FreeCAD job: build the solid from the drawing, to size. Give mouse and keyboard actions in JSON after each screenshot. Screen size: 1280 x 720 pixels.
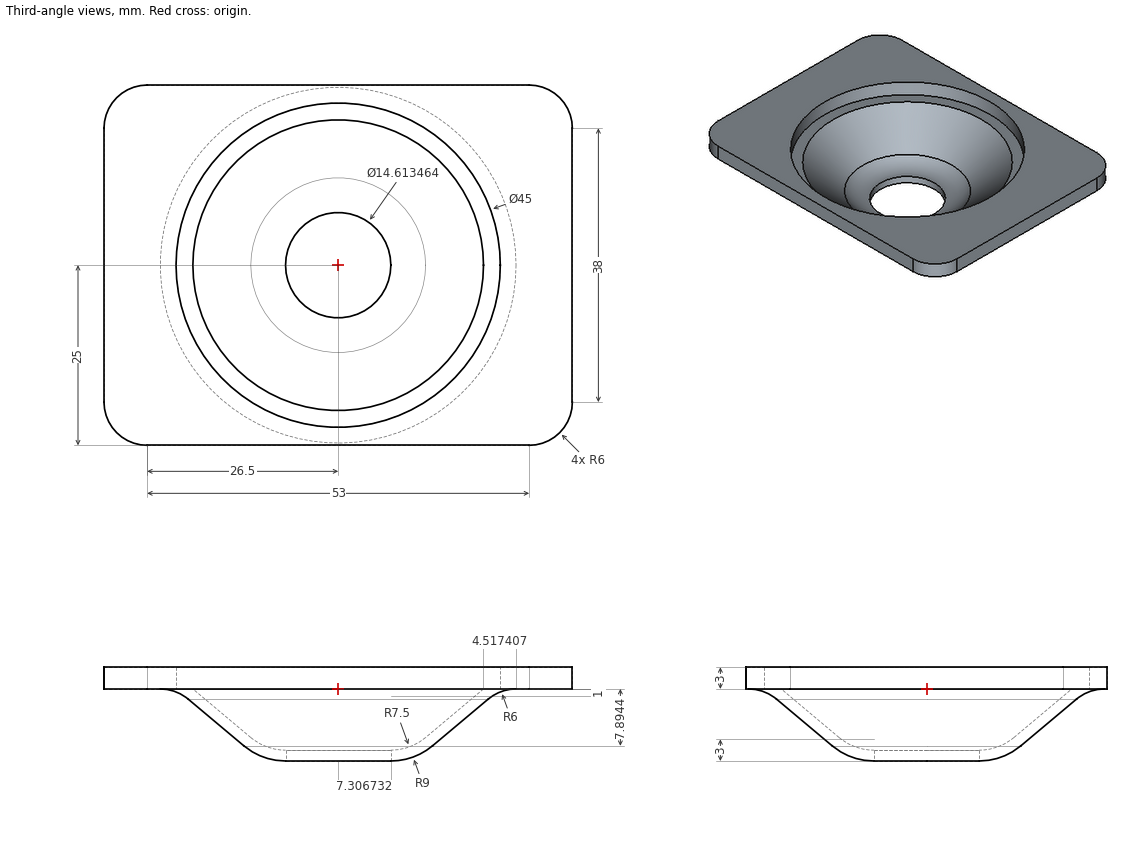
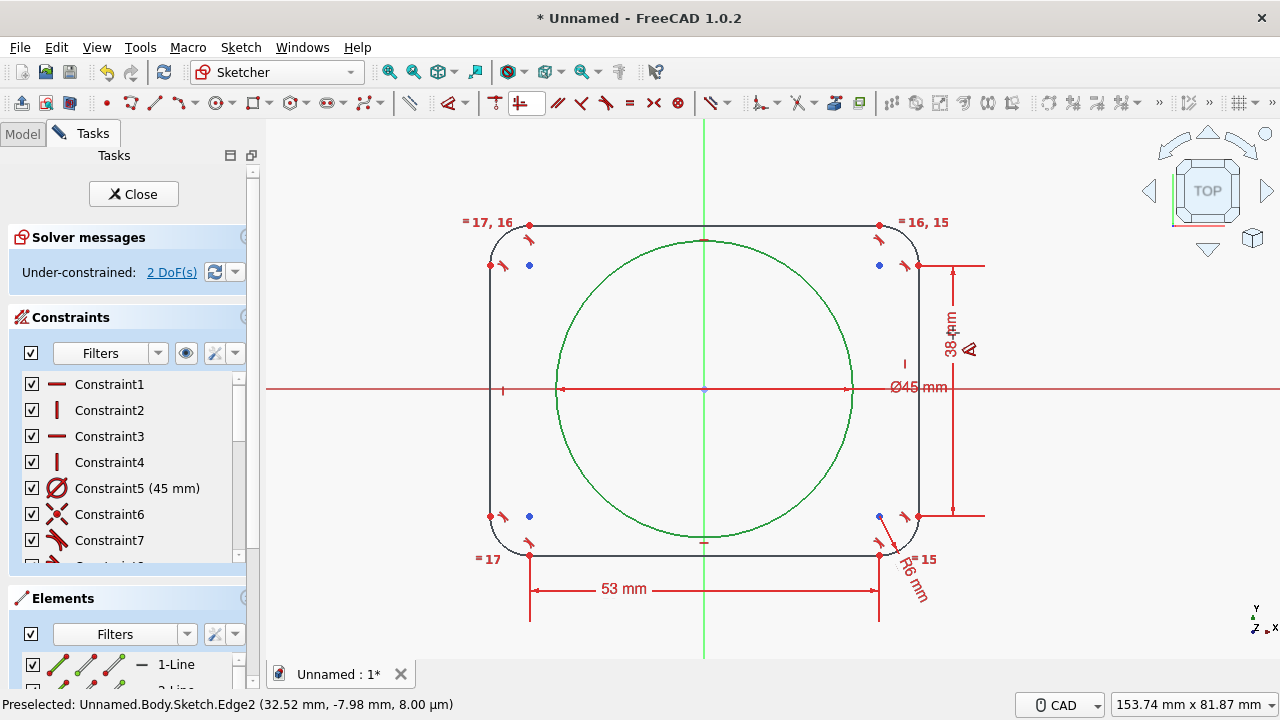
{"action": "left_click", "coordinate": [530, 556]}
{"action": "left_click", "coordinate": [738, 473]}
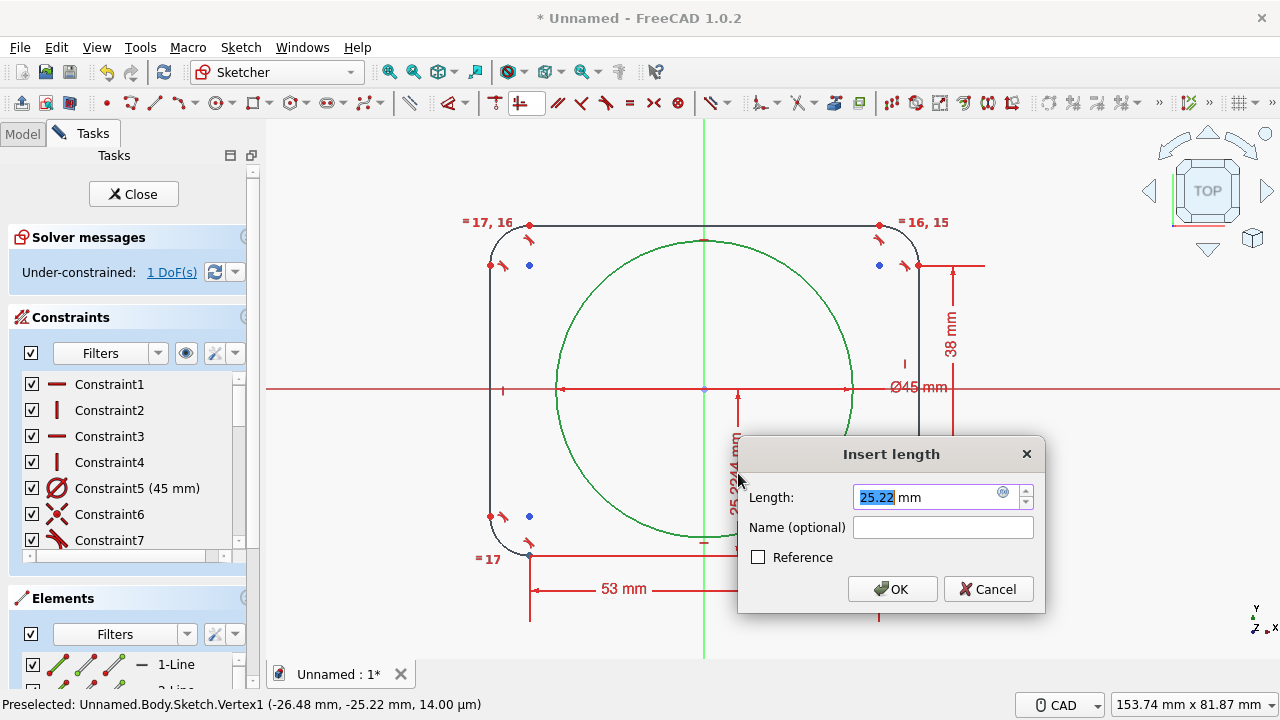
{"action": "type", "text": "25"}
{"action": "key", "text": "Return"}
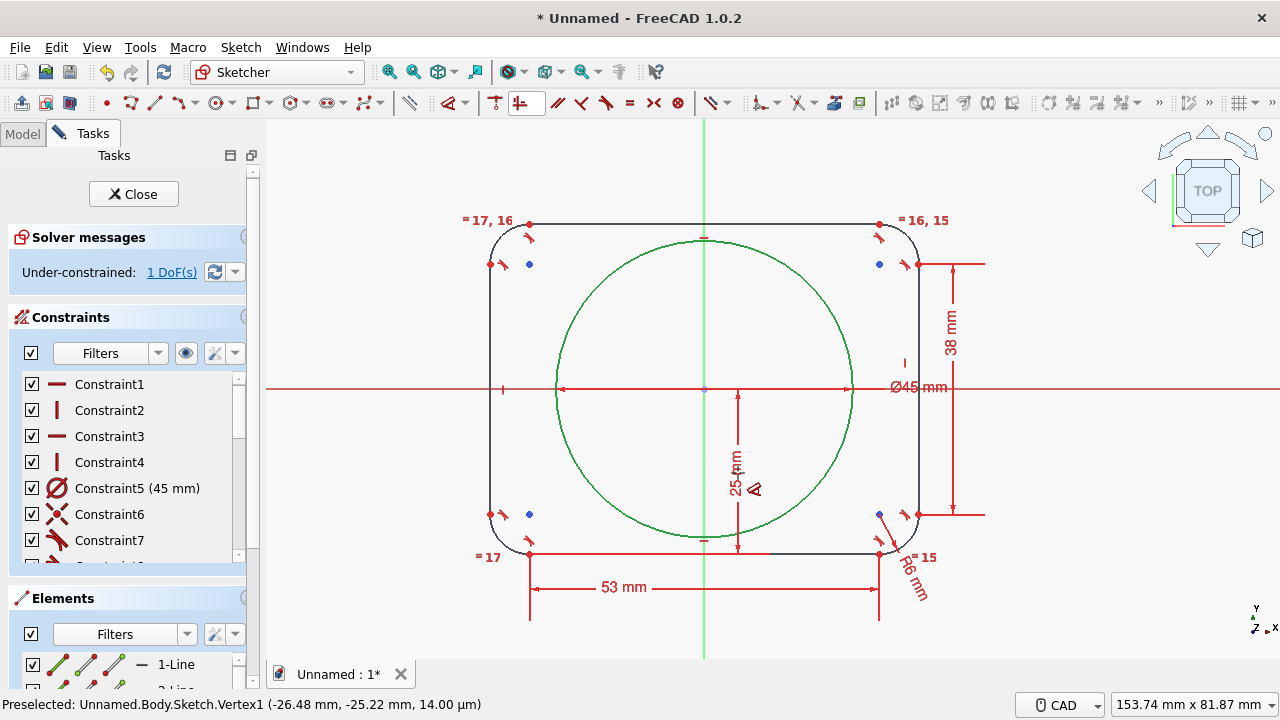
{"action": "left_click", "coordinate": [530, 554]}
{"action": "left_click", "coordinate": [617, 355]}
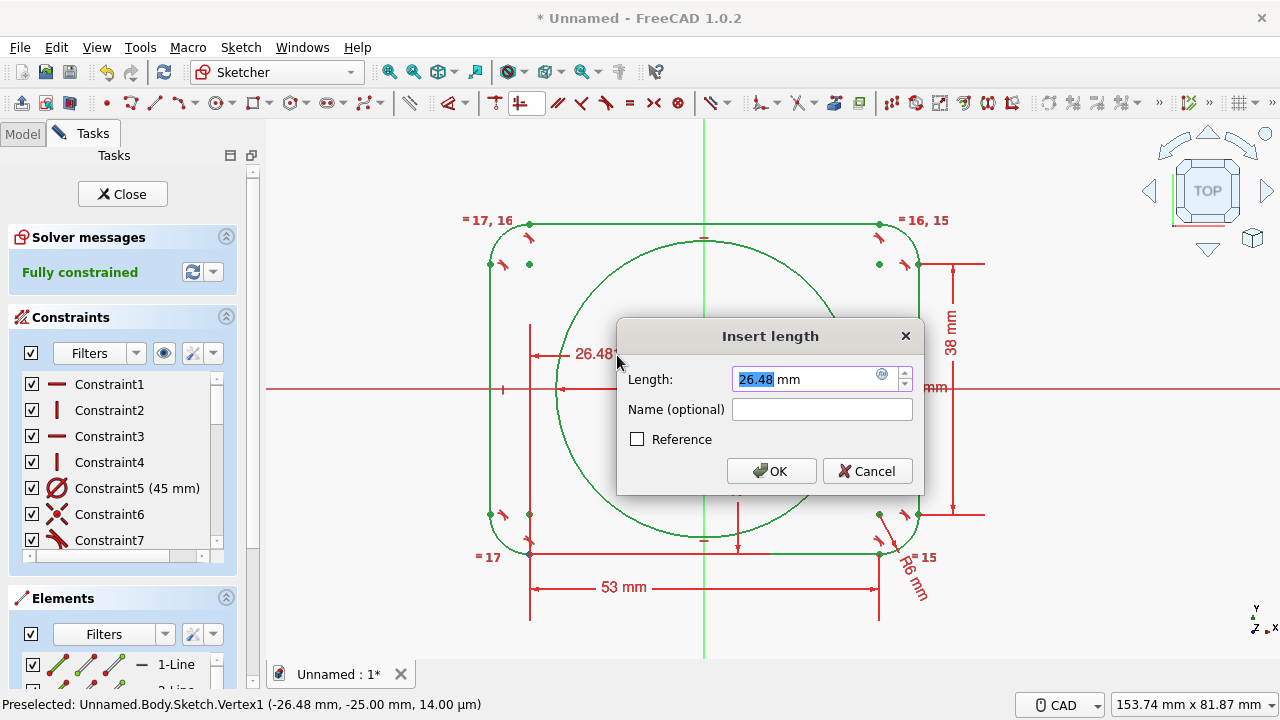
{"action": "type", "text": "26.5"}
{"action": "key", "text": "Return"}
{"action": "key", "text": "Escape"}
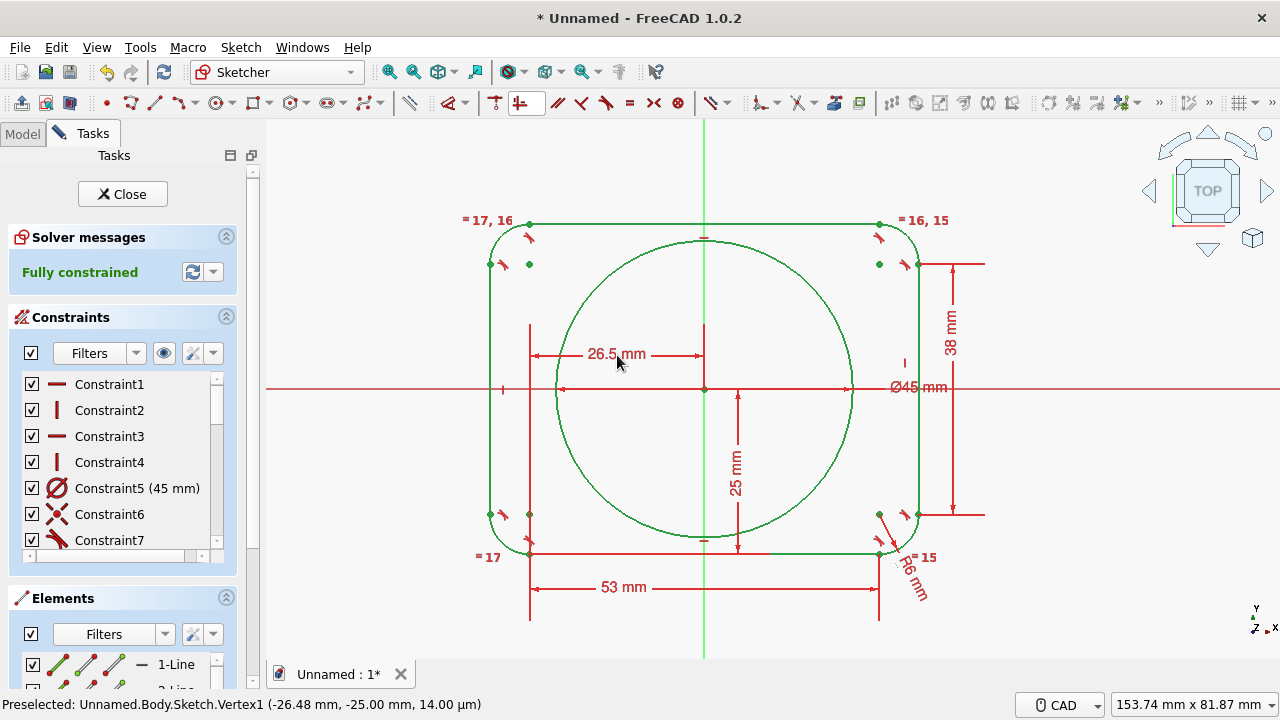
{"action": "left_click", "coordinate": [123, 194]}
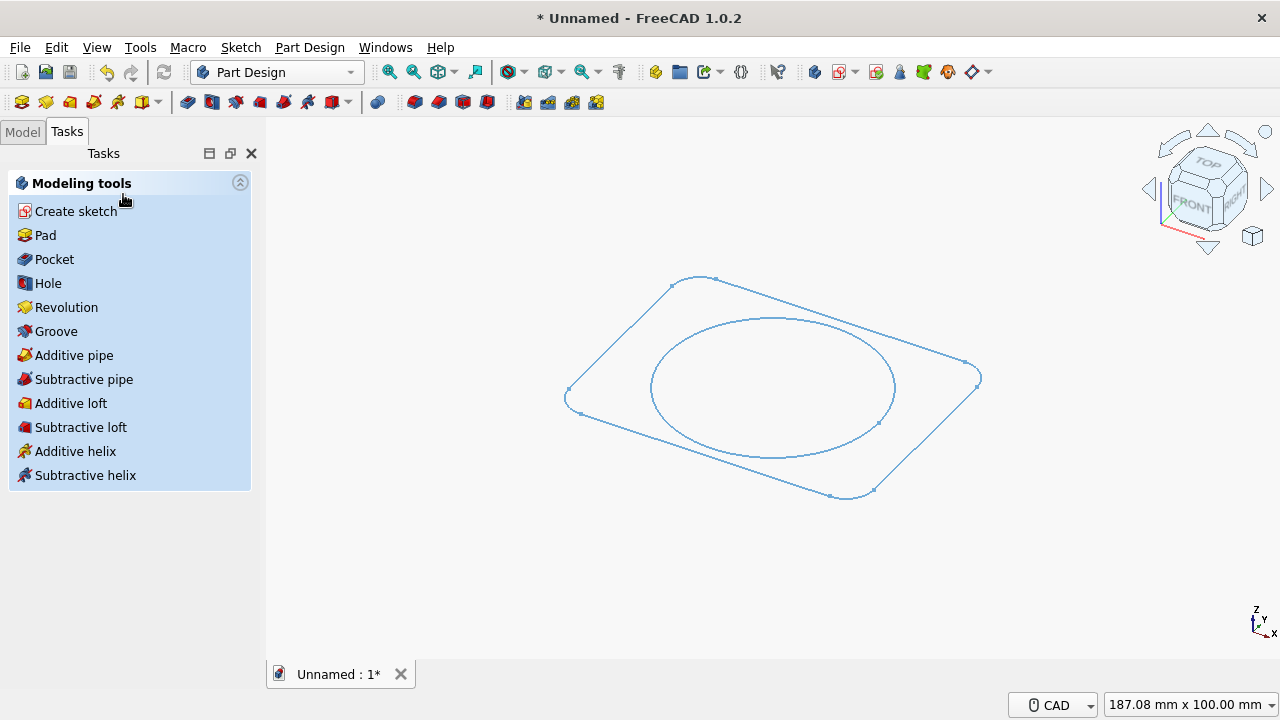
{"action": "left_click", "coordinate": [22, 102]}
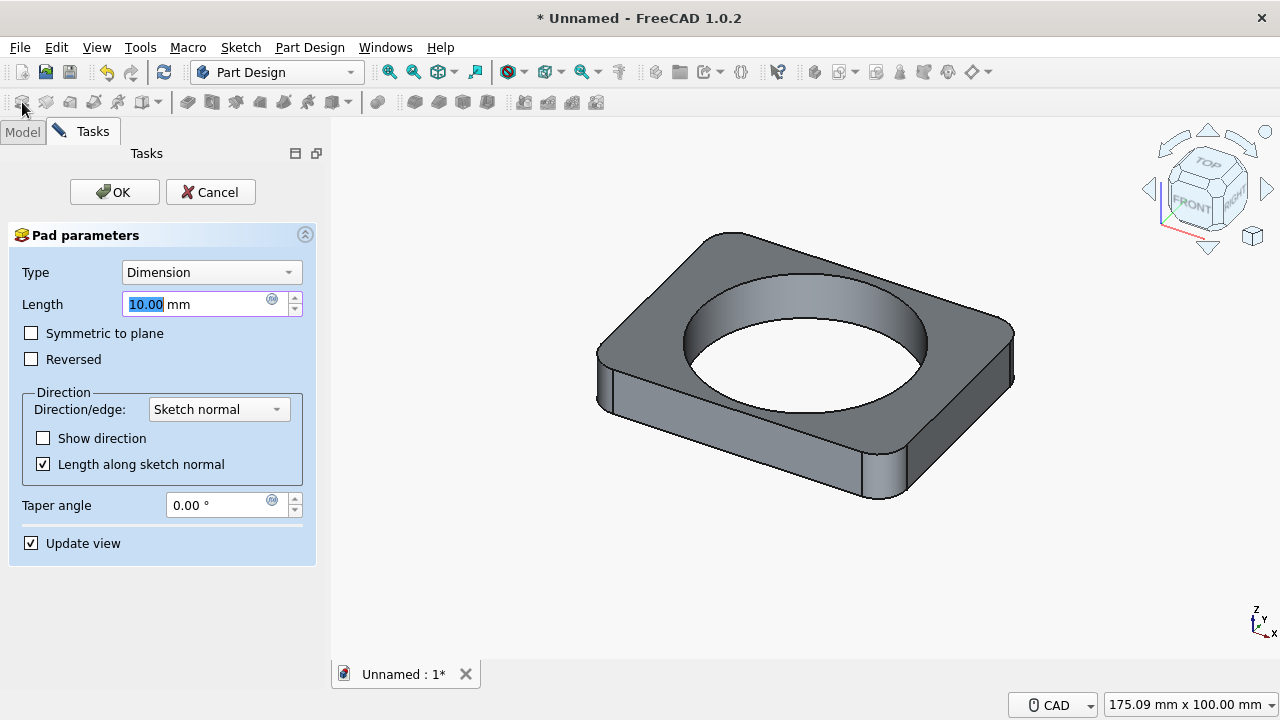
{"action": "type", "text": "3"}
{"action": "key", "text": "Tab"}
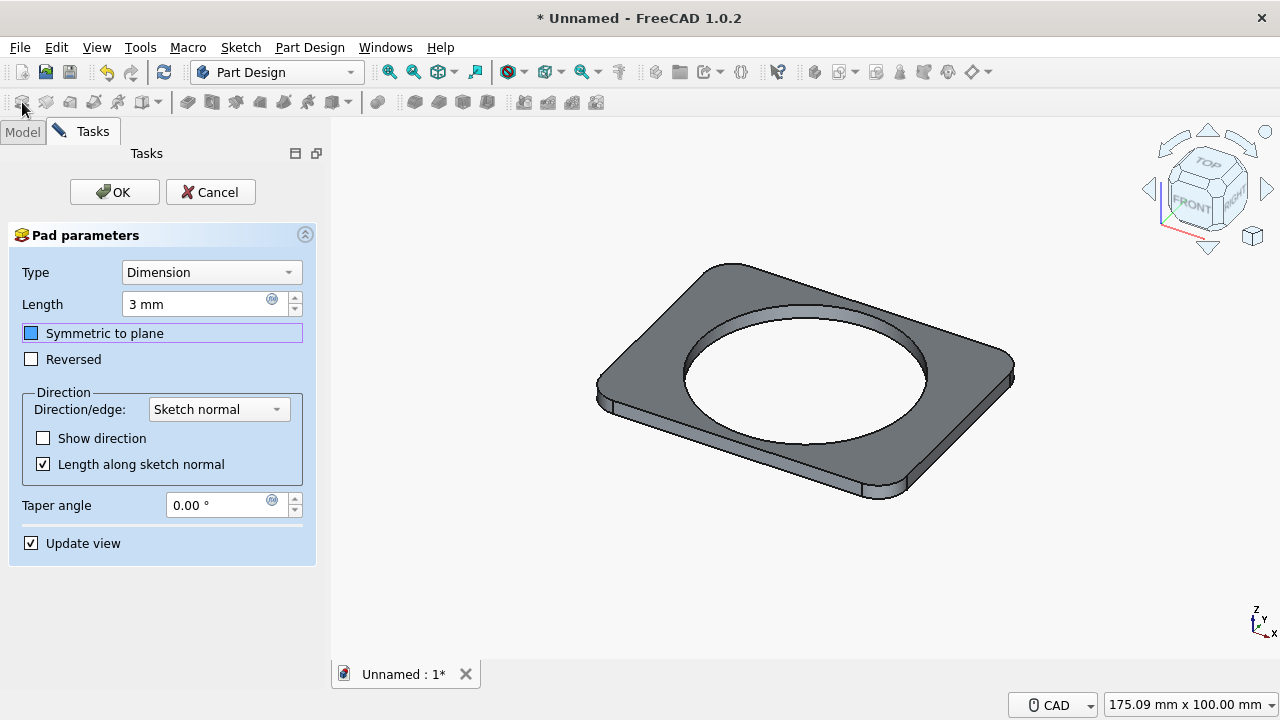
{"action": "left_click", "coordinate": [115, 192]}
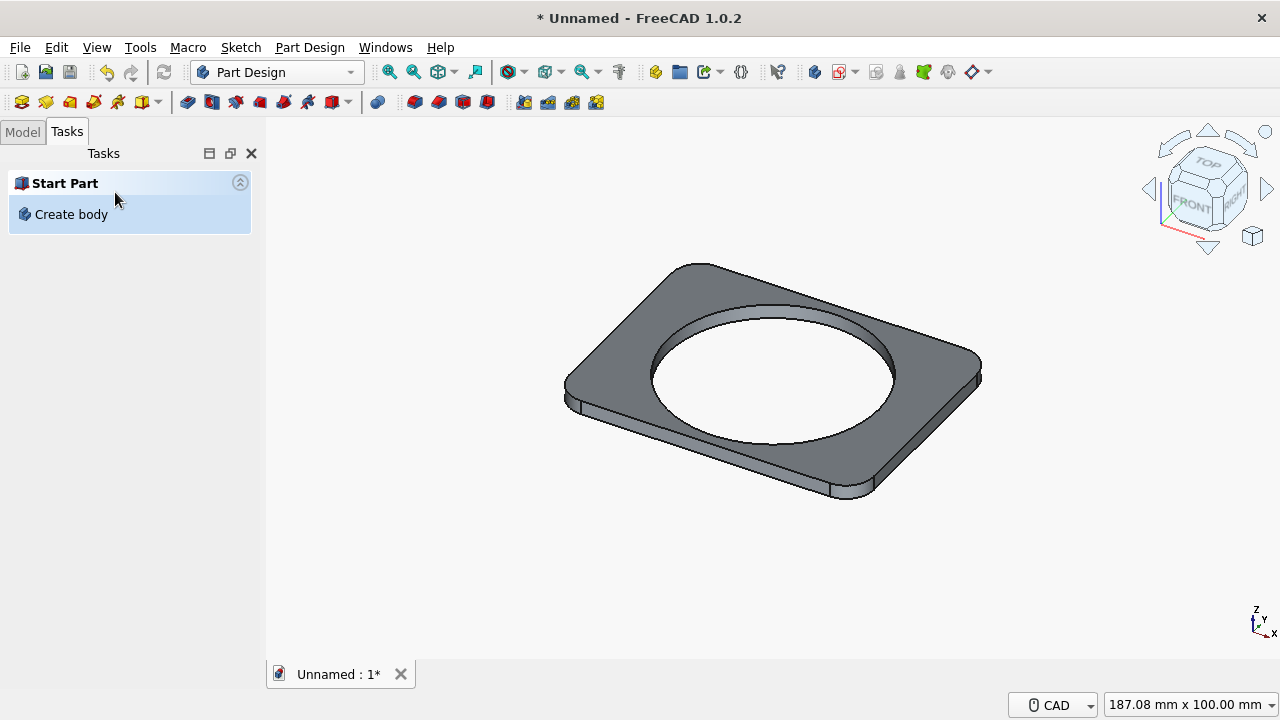
{"action": "left_click", "coordinate": [840, 72]}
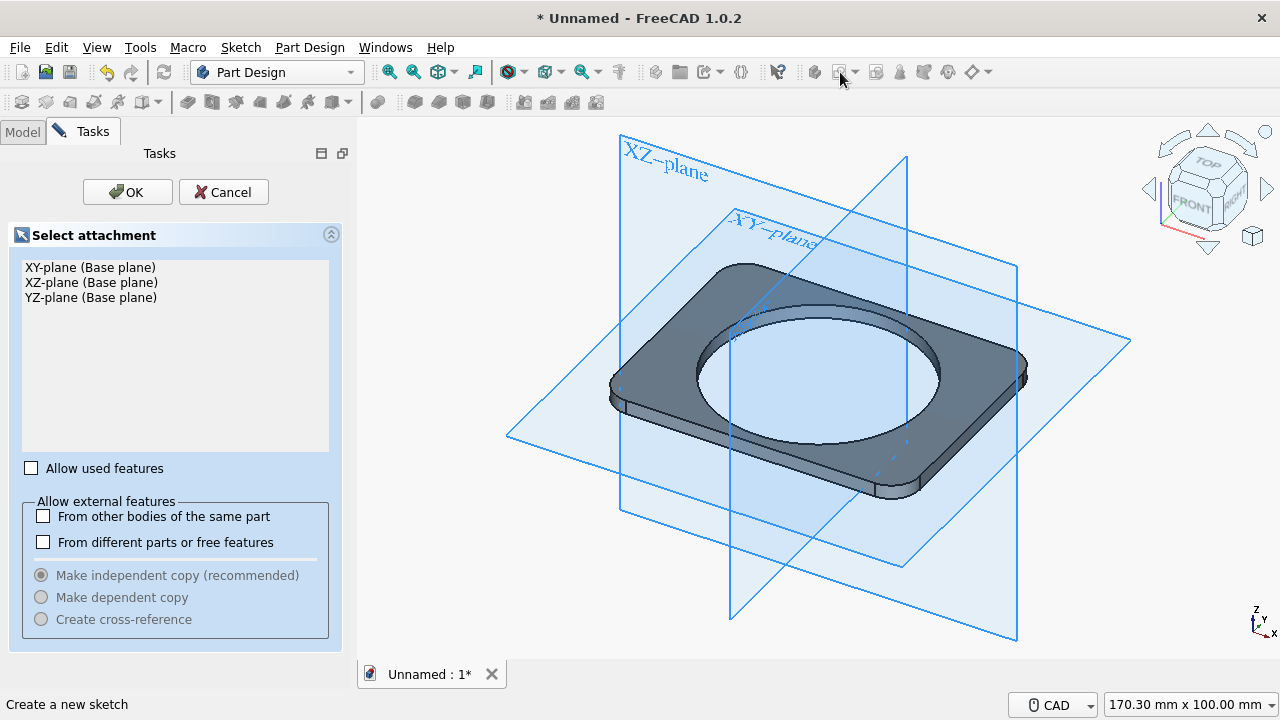
{"action": "left_click", "coordinate": [82, 282]}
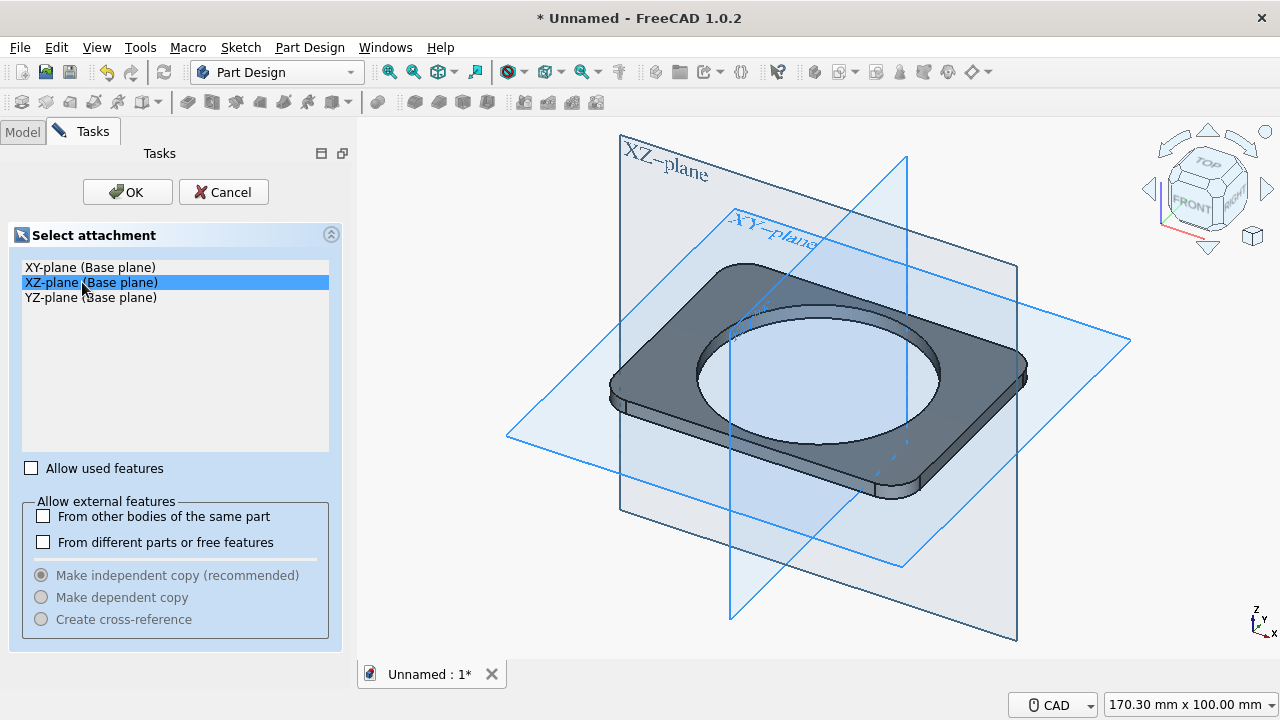
{"action": "left_click", "coordinate": [128, 192]}